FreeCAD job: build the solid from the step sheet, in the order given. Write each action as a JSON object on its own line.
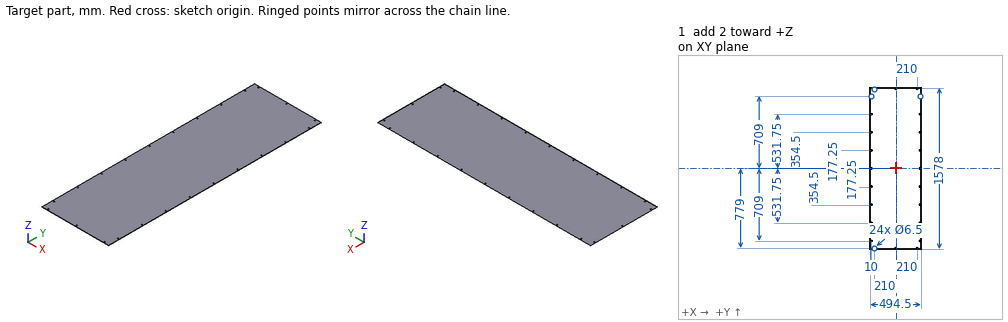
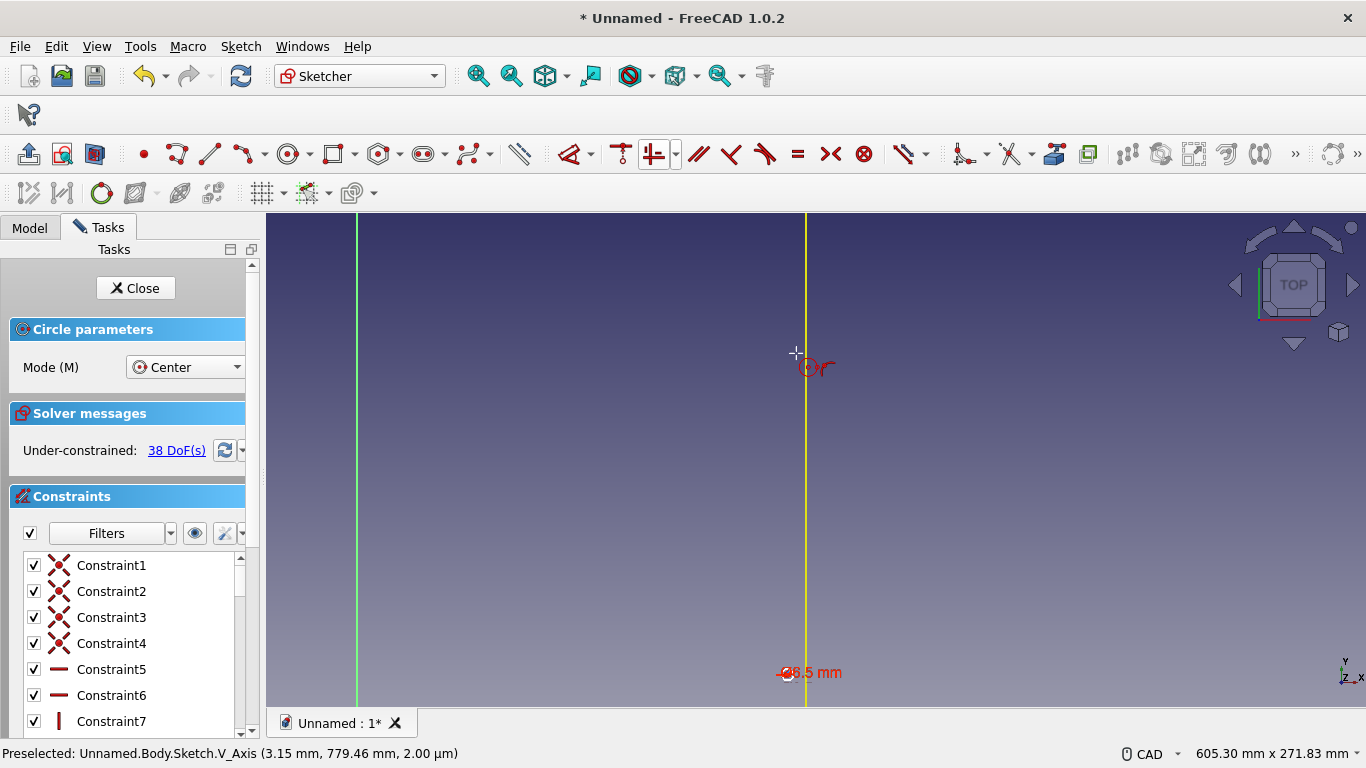
{"action": "left_click", "coordinate": [788, 352]}
{"action": "mouse_move", "coordinate": [784, 348]}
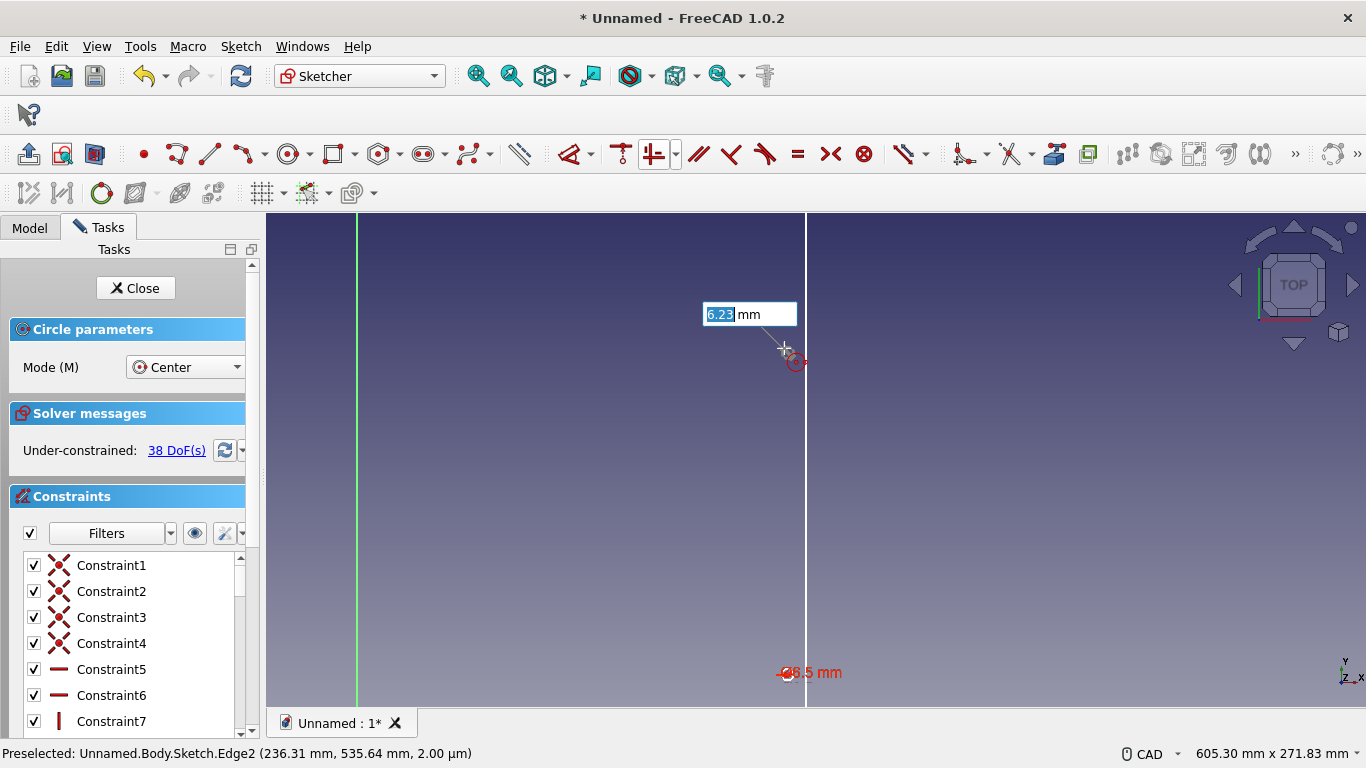
{"action": "type", "text": "6.5"}
{"action": "key", "text": "Return"}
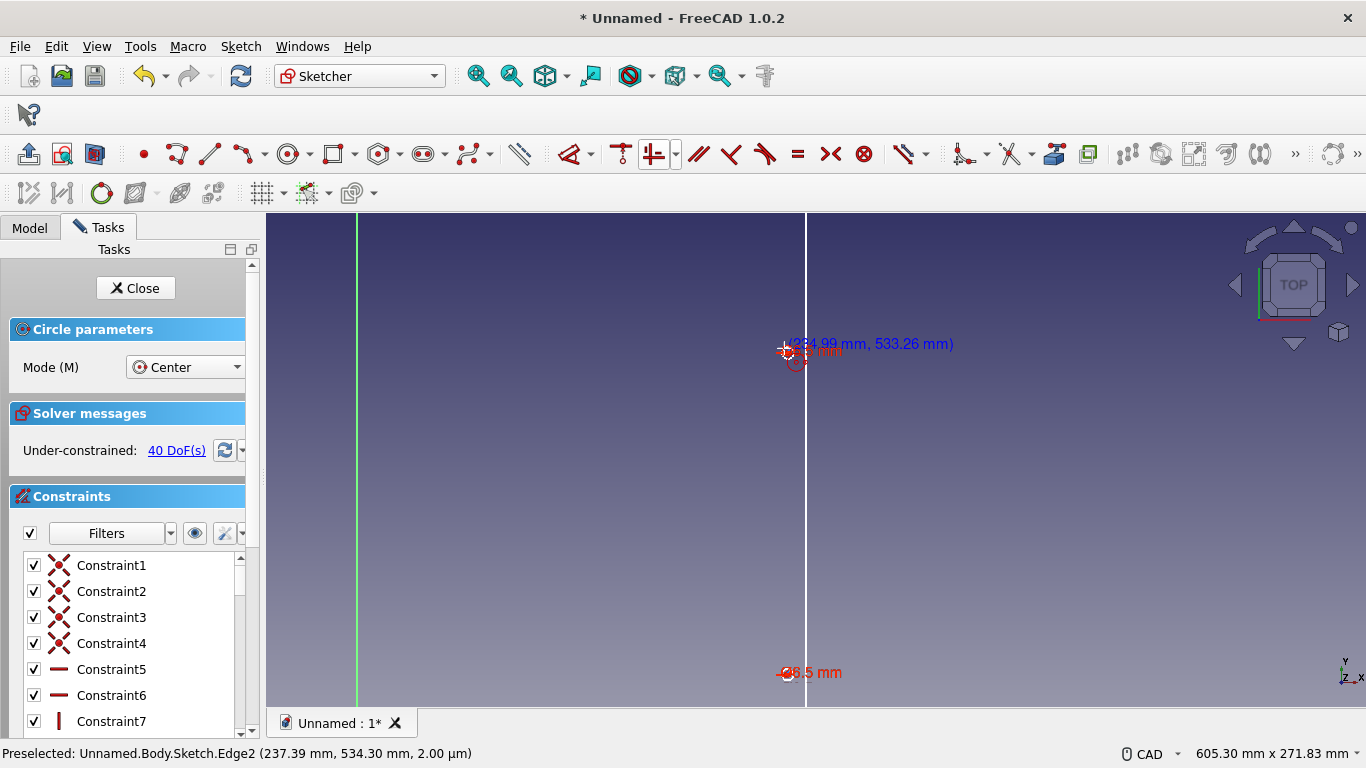
{"action": "scroll", "coordinate": [796, 353], "scroll_direction": "down", "scroll_amount": 11}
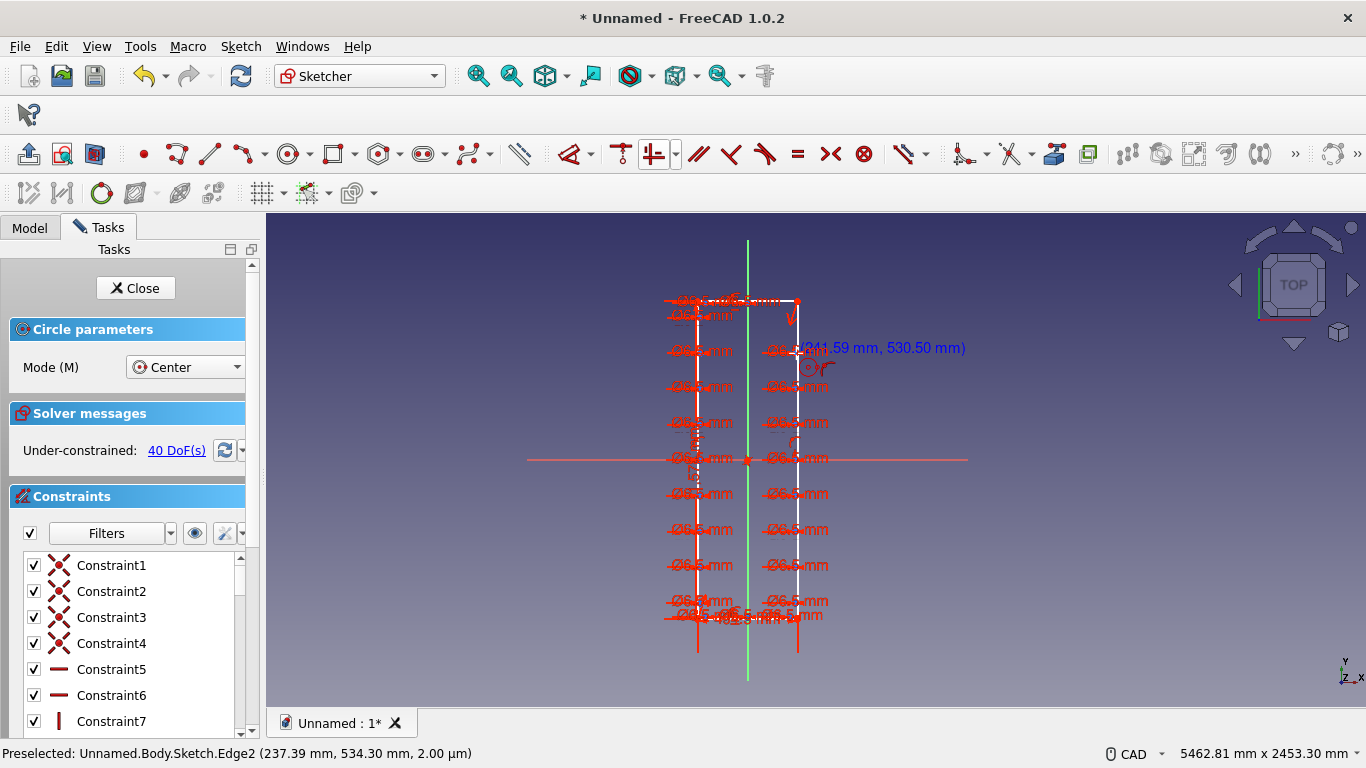
{"action": "scroll", "coordinate": [790, 303], "scroll_direction": "up", "scroll_amount": 18}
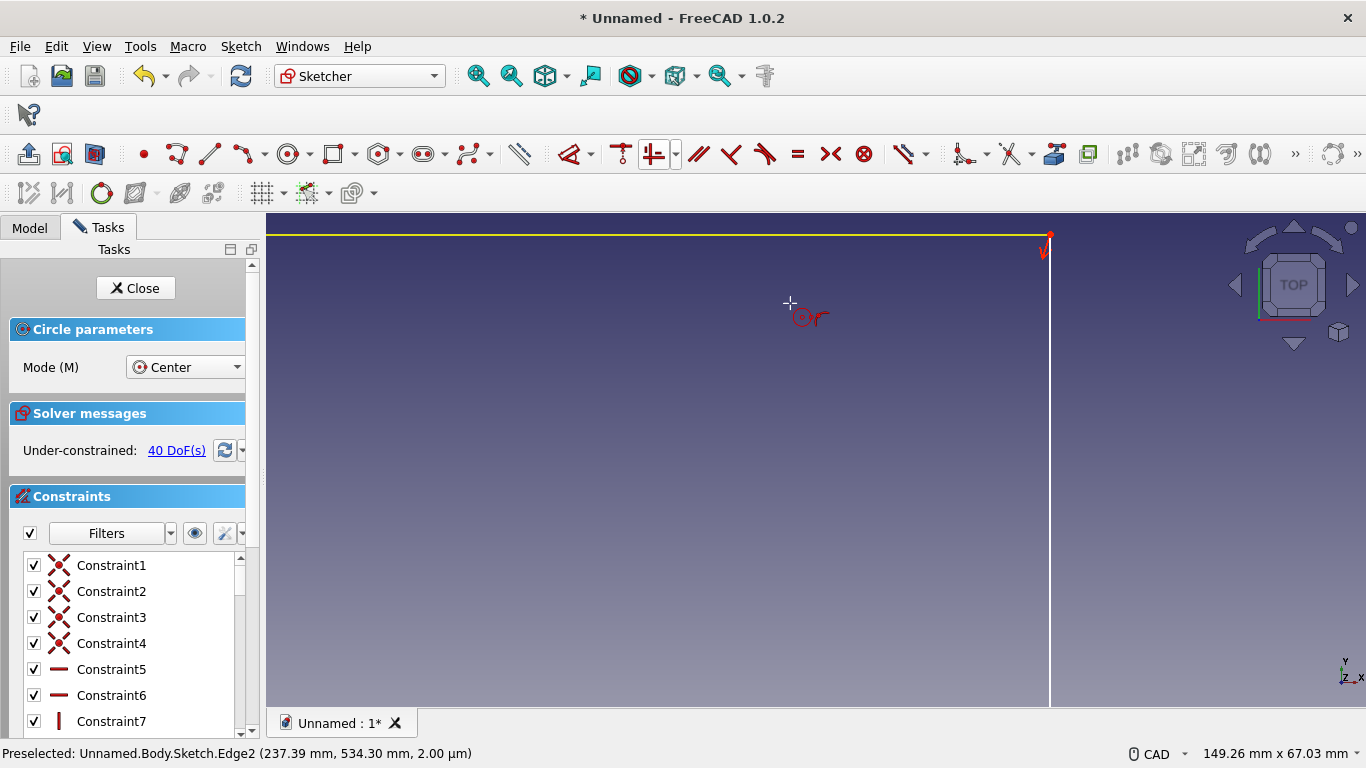
{"action": "scroll", "coordinate": [790, 303], "scroll_direction": "down", "scroll_amount": 18}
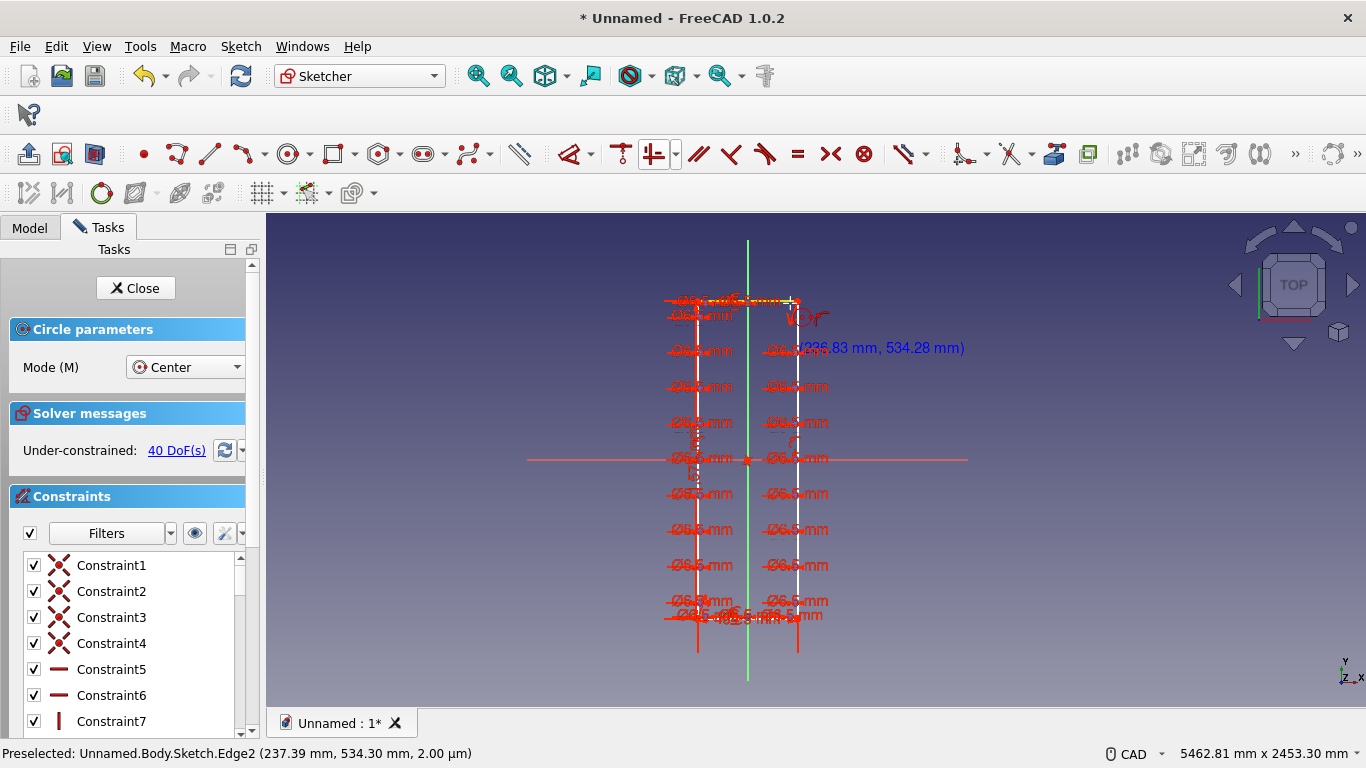
{"action": "scroll", "coordinate": [790, 303], "scroll_direction": "up", "scroll_amount": 11}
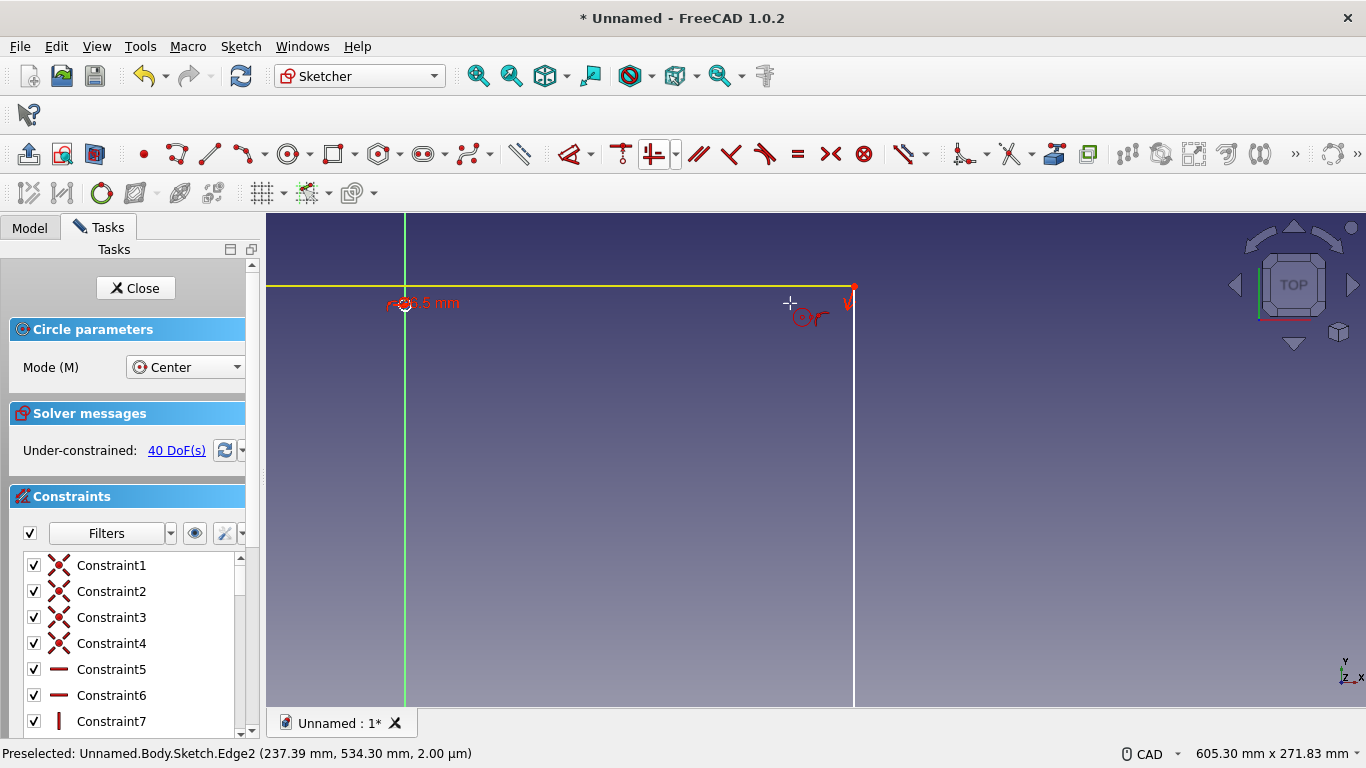
{"action": "left_click", "coordinate": [787, 304]}
{"action": "mouse_move", "coordinate": [791, 309]}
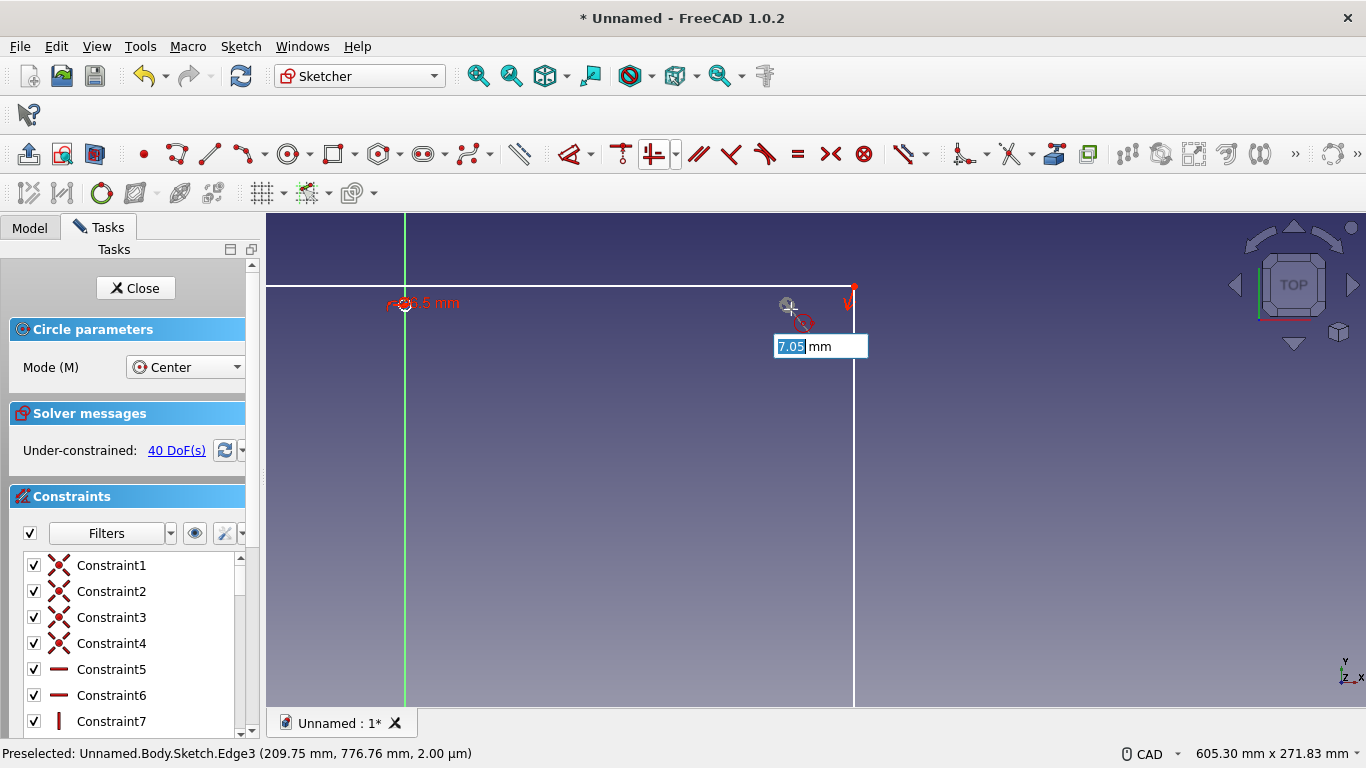
{"action": "type", "text": "6.5"}
{"action": "key", "text": "Return"}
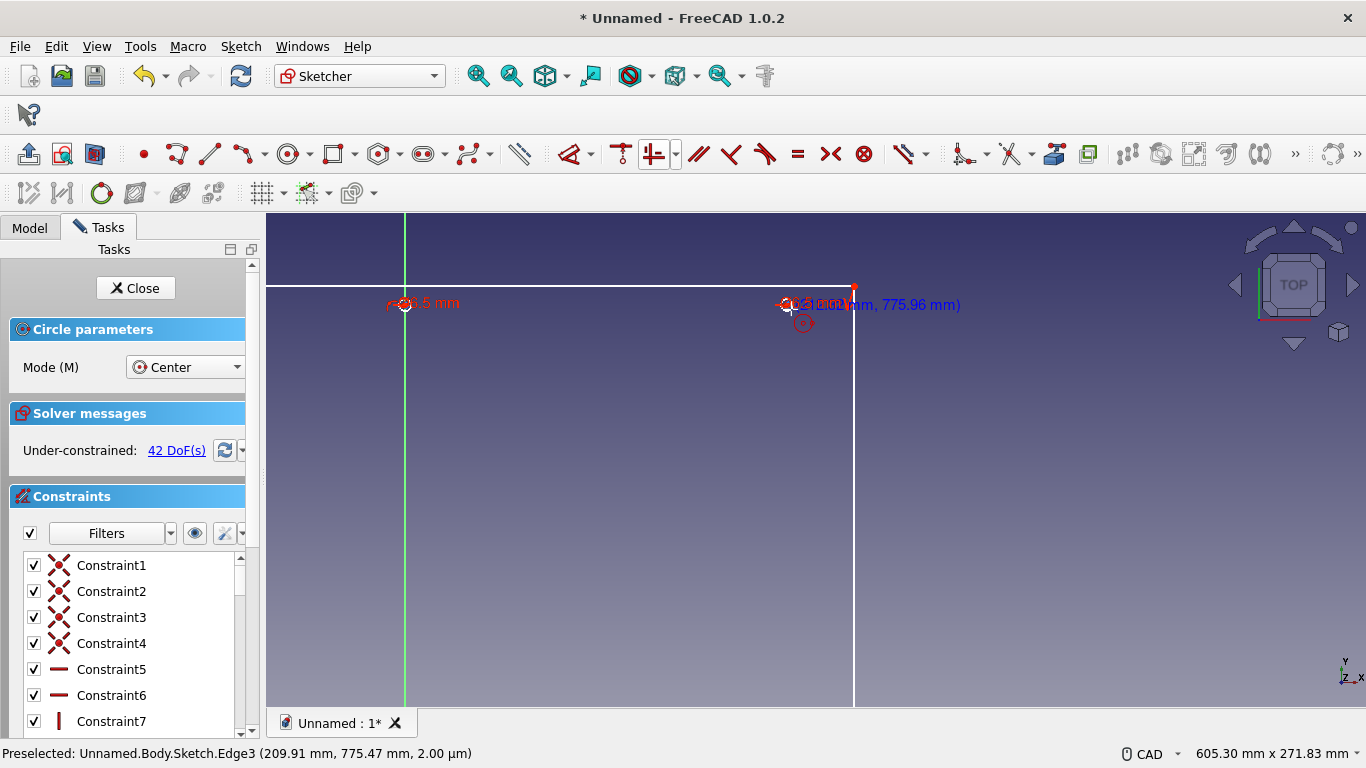
{"action": "scroll", "coordinate": [836, 432], "scroll_direction": "up", "scroll_amount": 7}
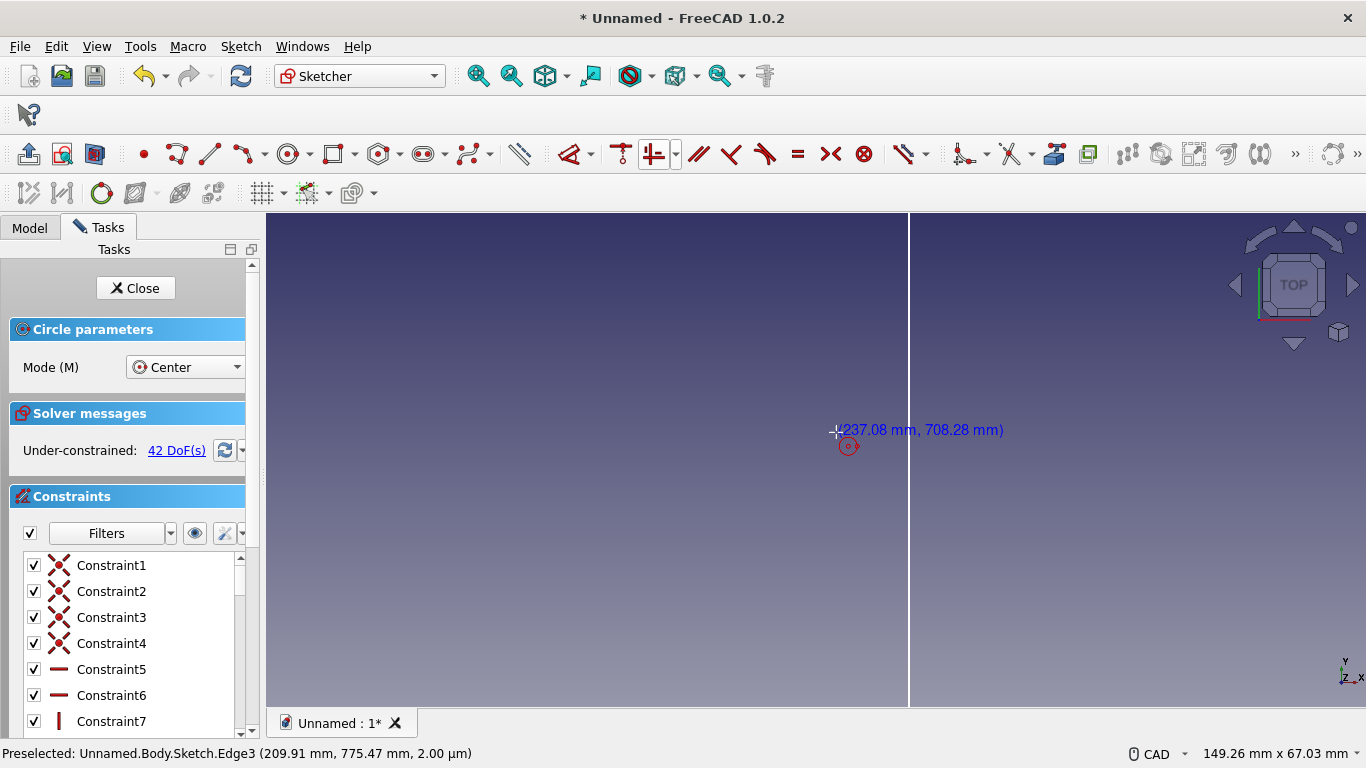
{"action": "scroll", "coordinate": [794, 314], "scroll_direction": "down", "scroll_amount": 18}